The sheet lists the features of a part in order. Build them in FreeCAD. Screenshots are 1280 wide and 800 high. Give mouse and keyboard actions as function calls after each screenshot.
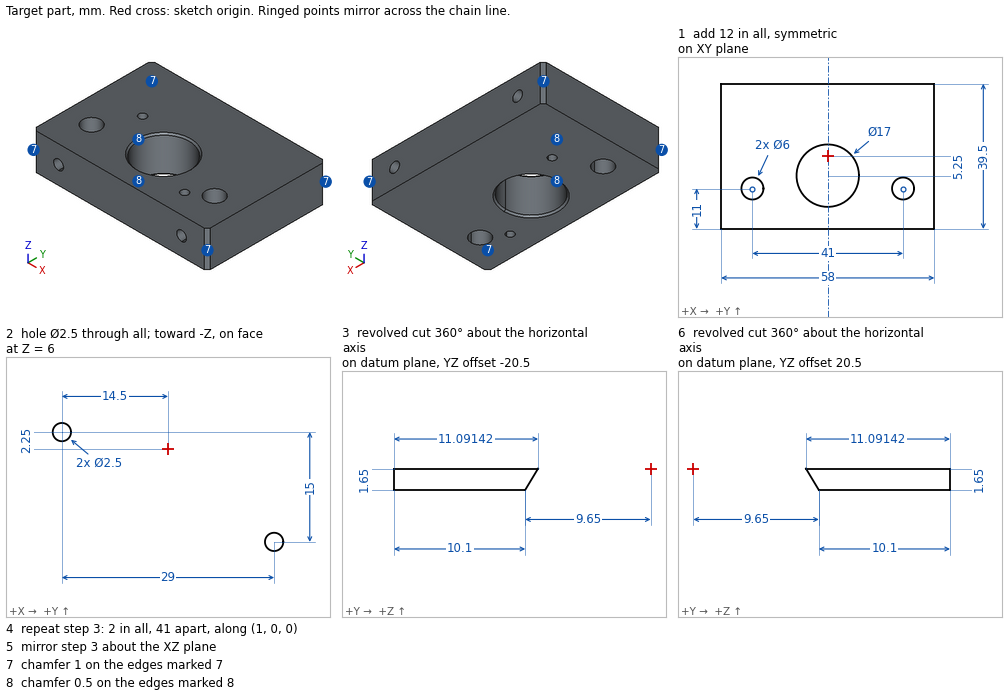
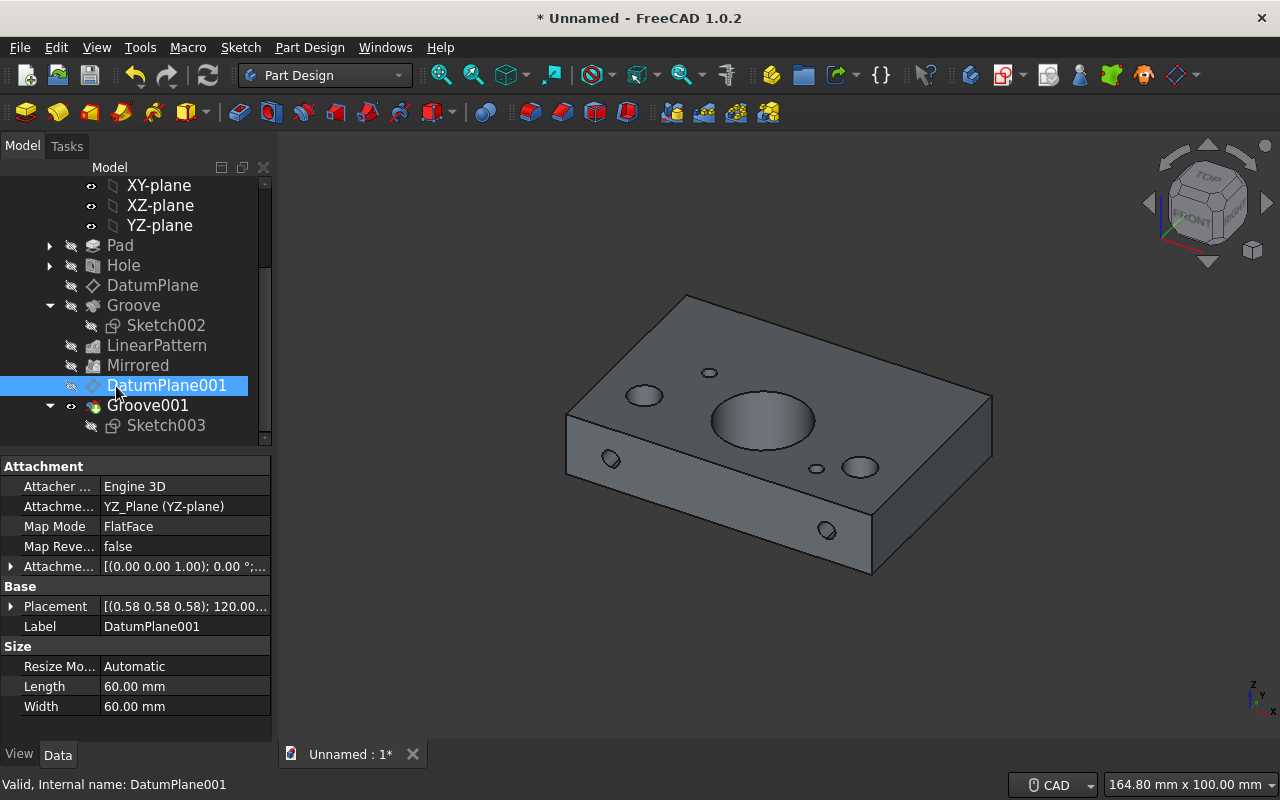
click(872, 544)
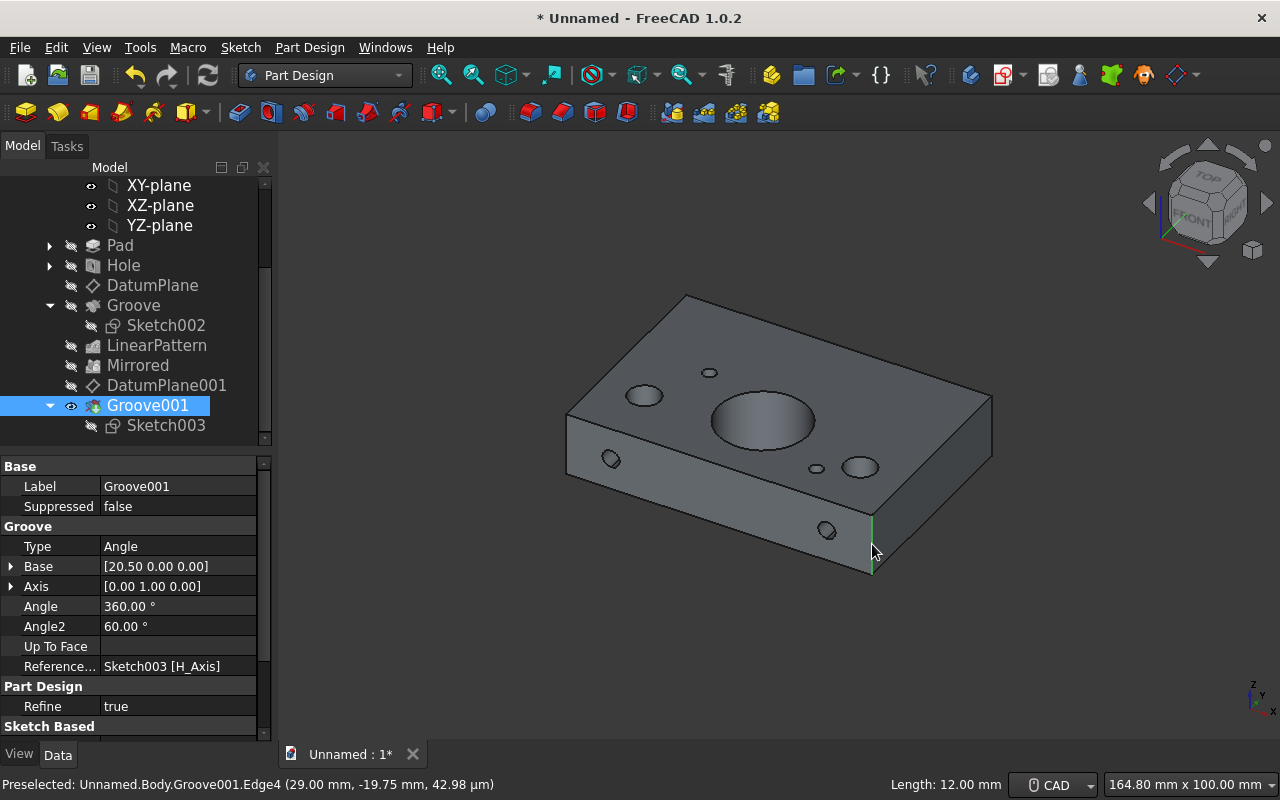
key(0)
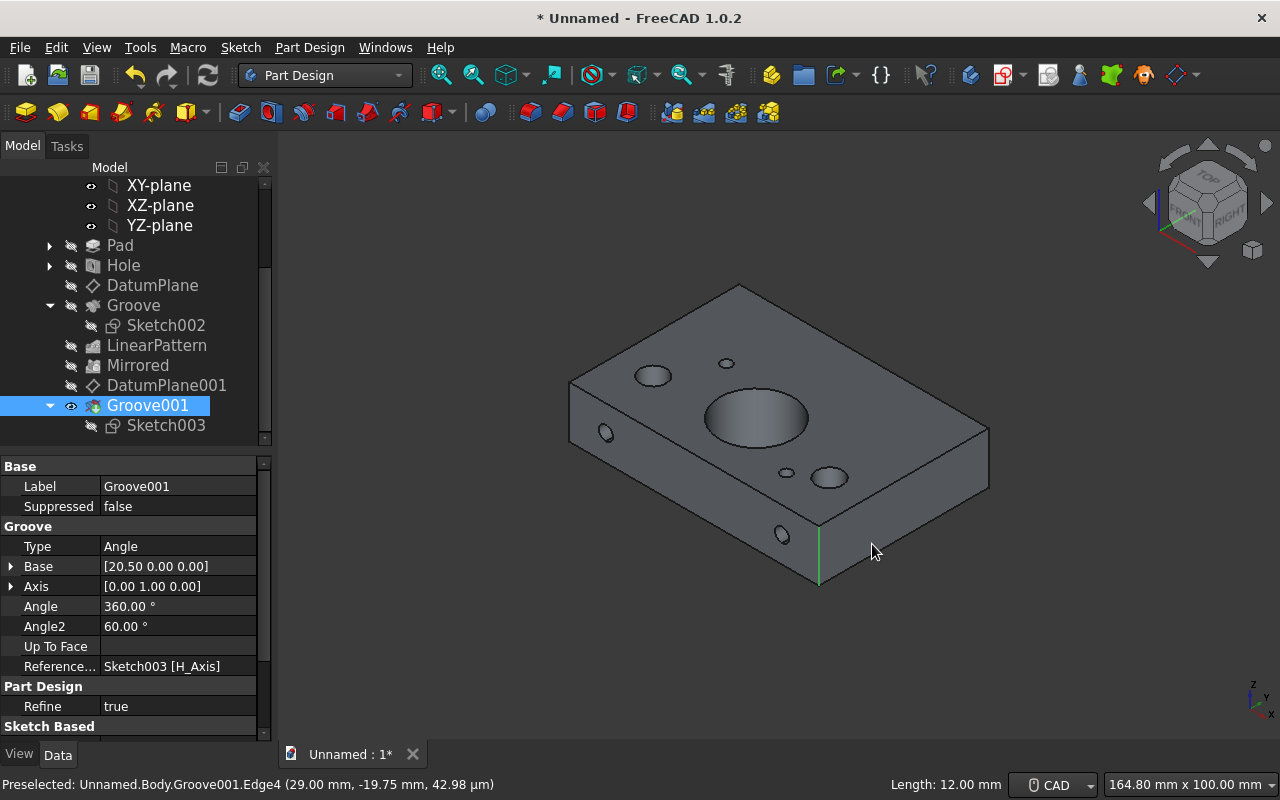
key(2)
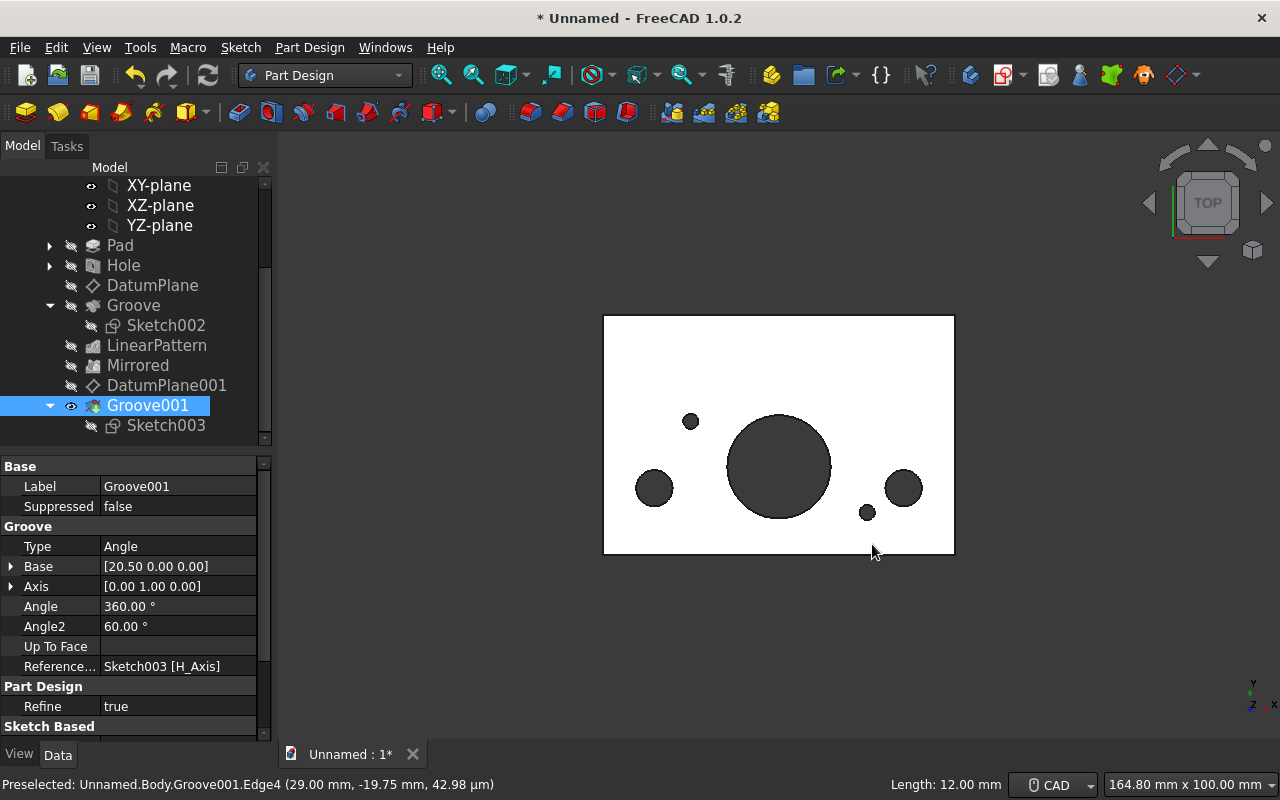
key(v)
key(f)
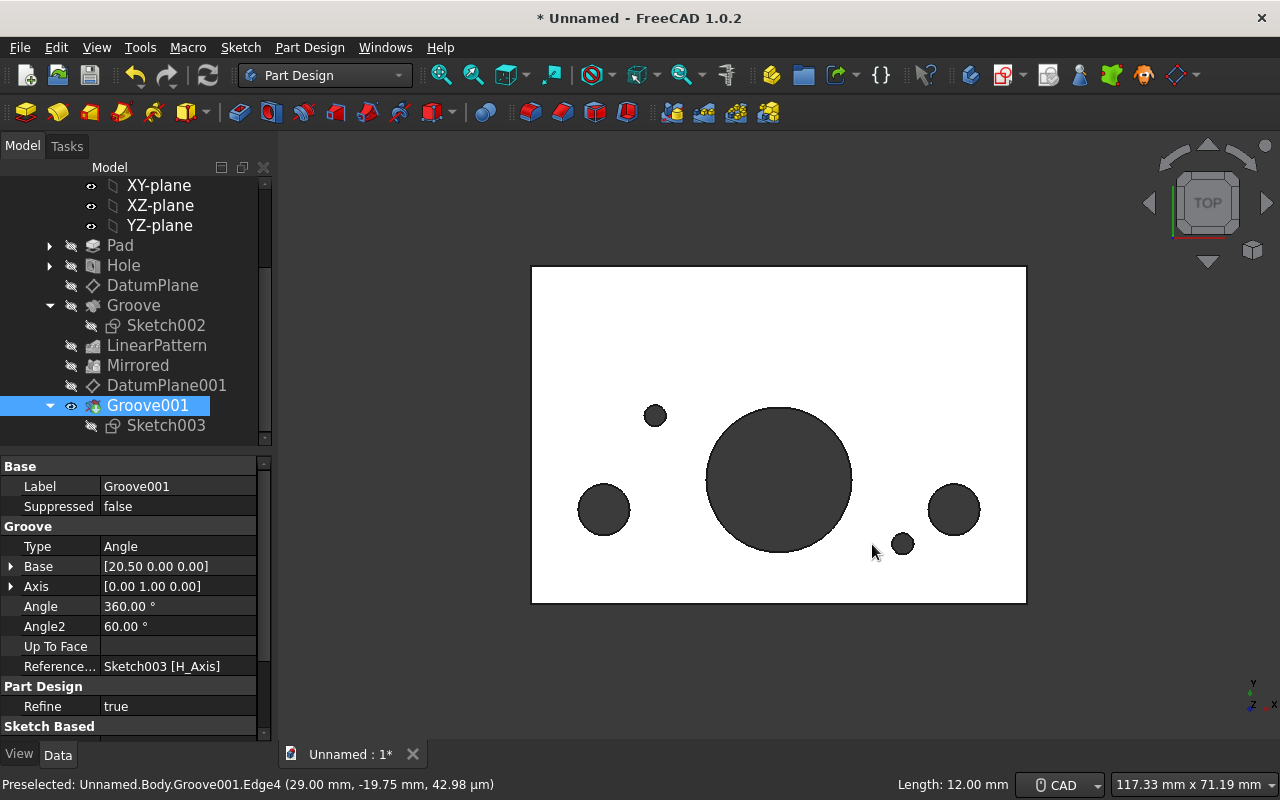
key(1)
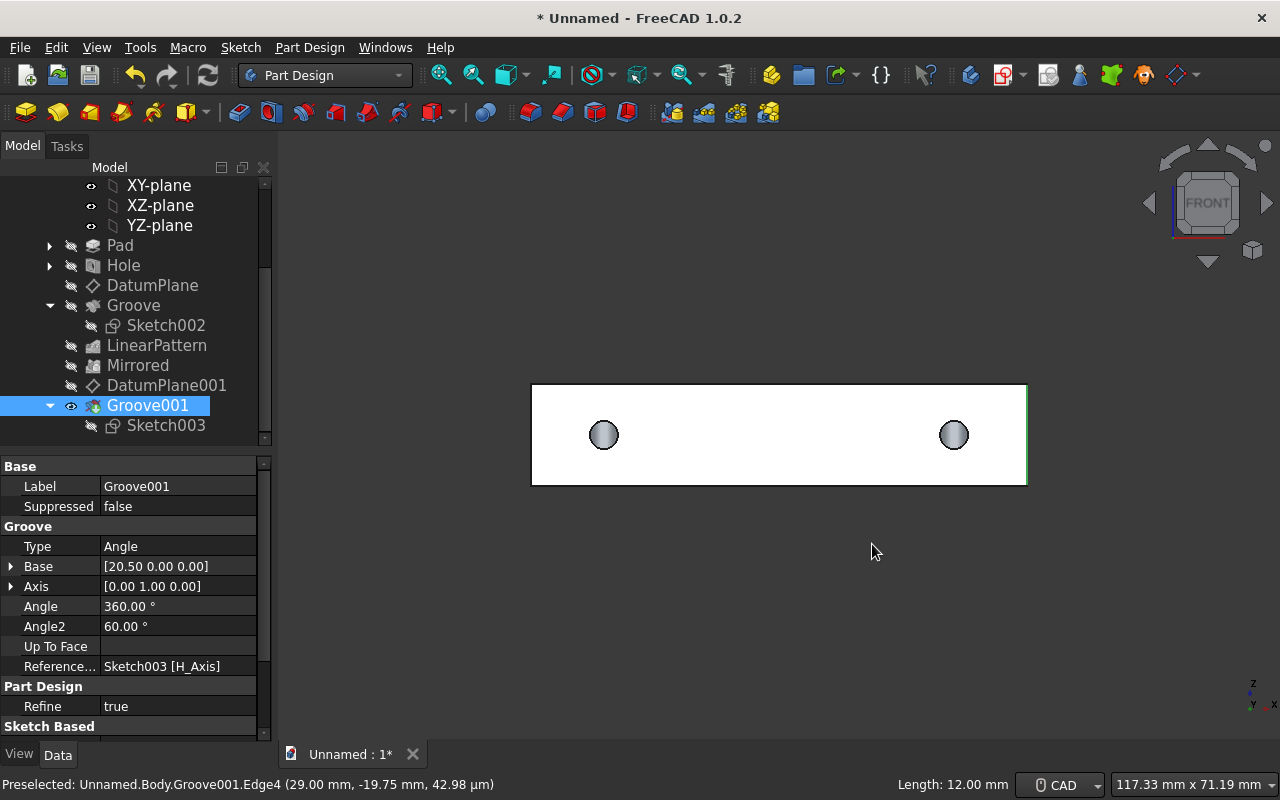
click(531, 434, ctrl)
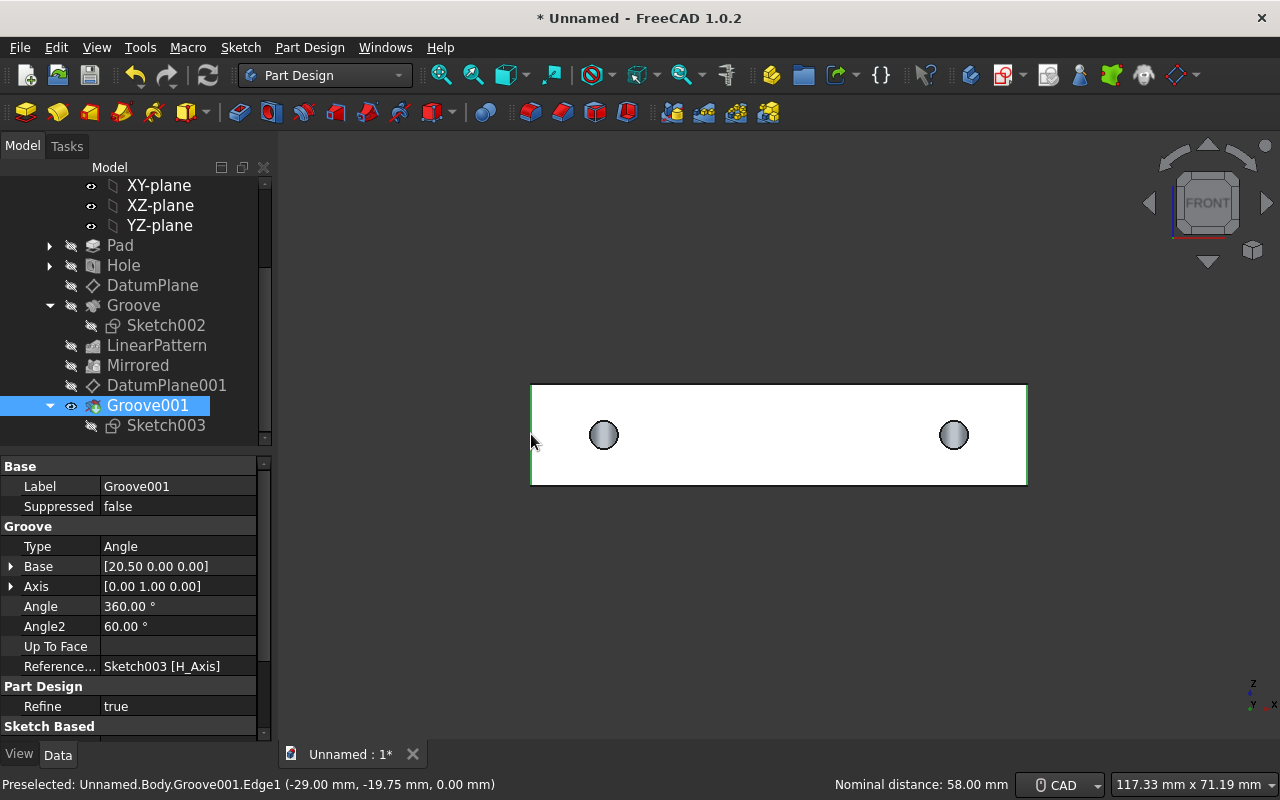
key(3)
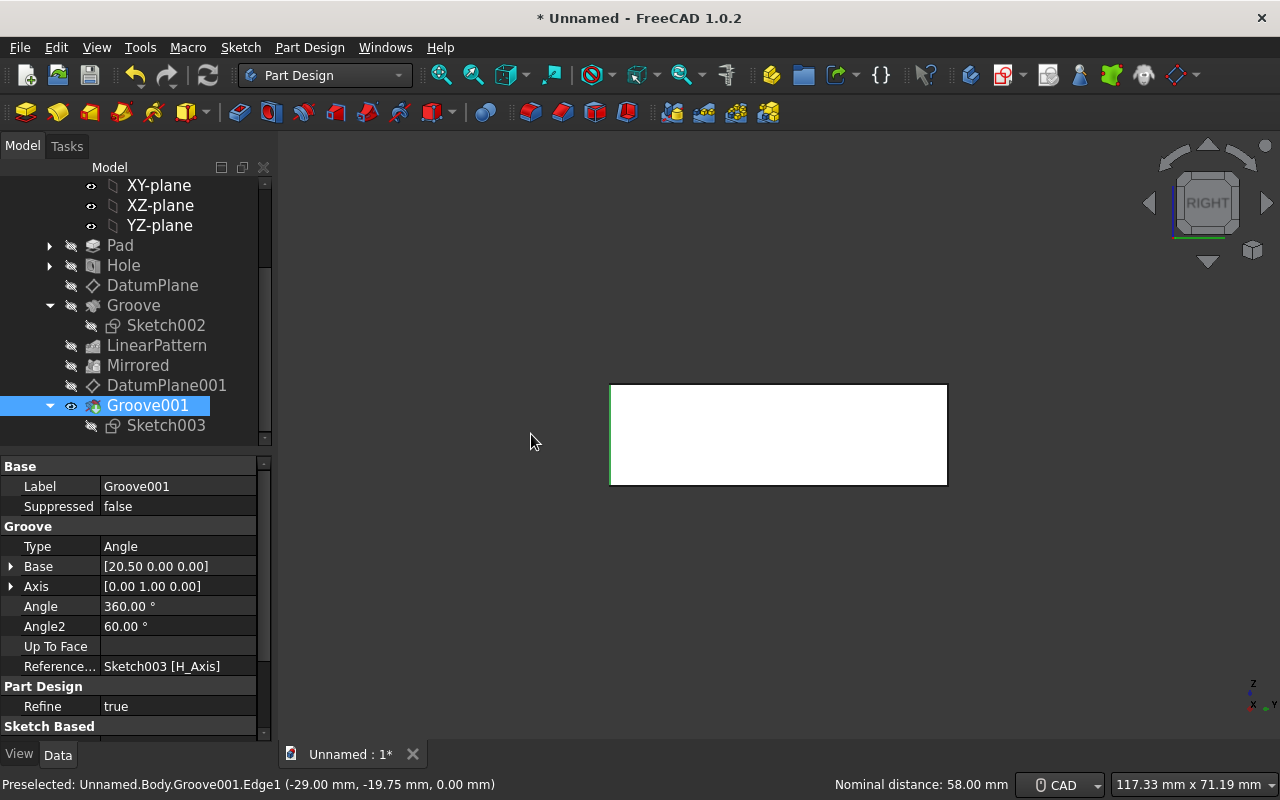
key(v)
key(f)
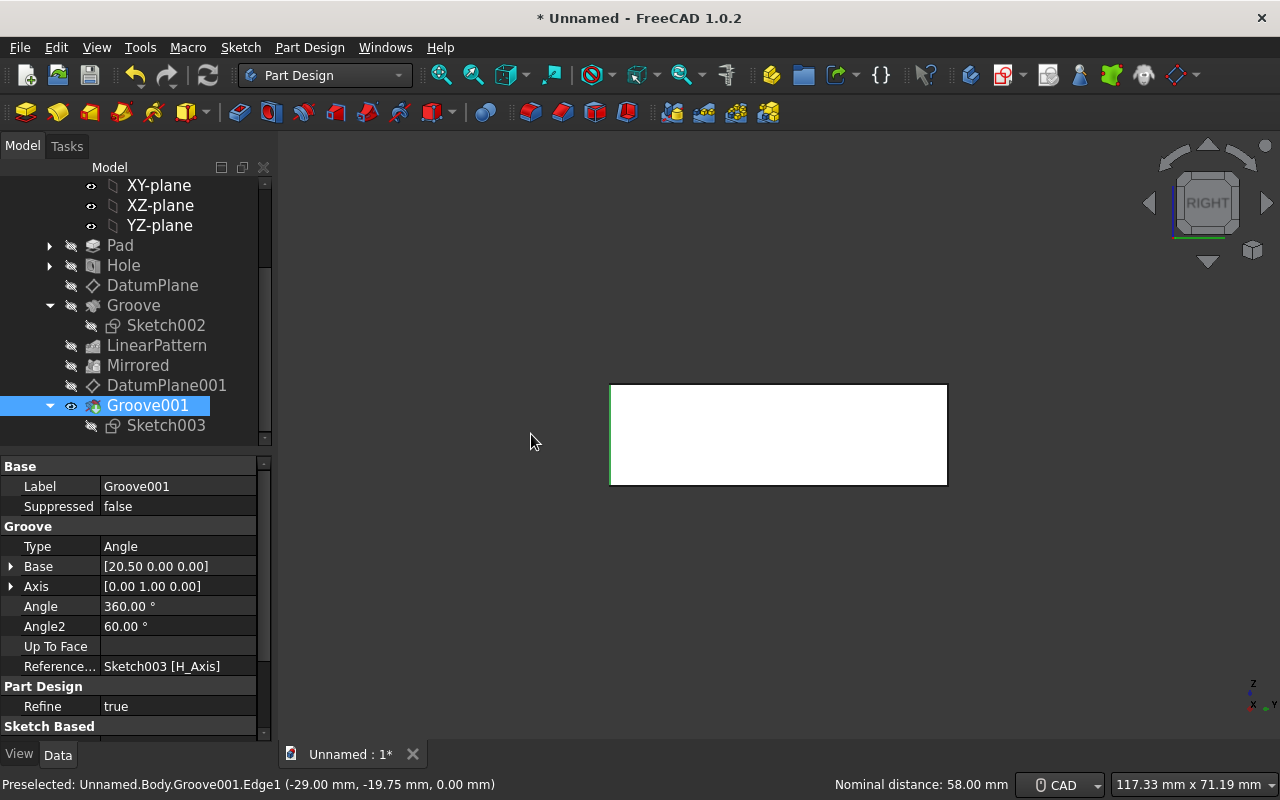
click(948, 434, ctrl)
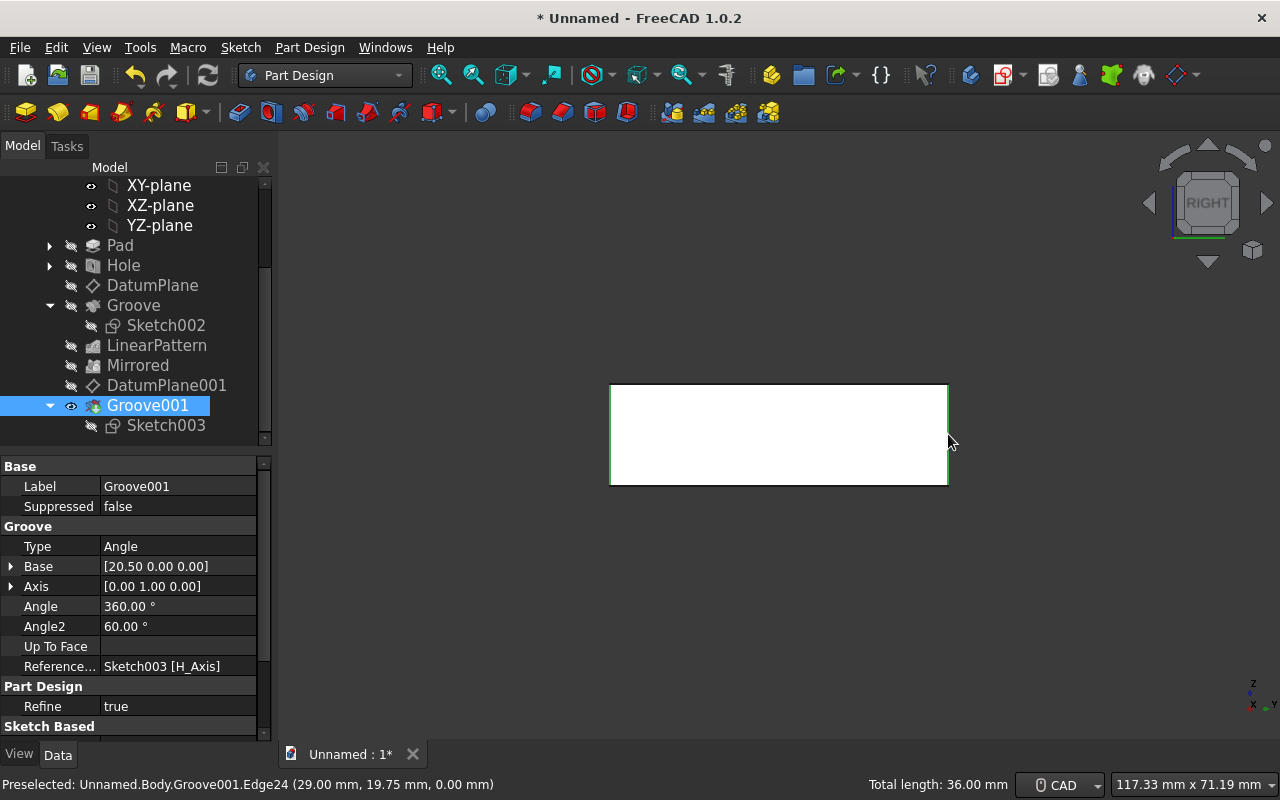
key(5)